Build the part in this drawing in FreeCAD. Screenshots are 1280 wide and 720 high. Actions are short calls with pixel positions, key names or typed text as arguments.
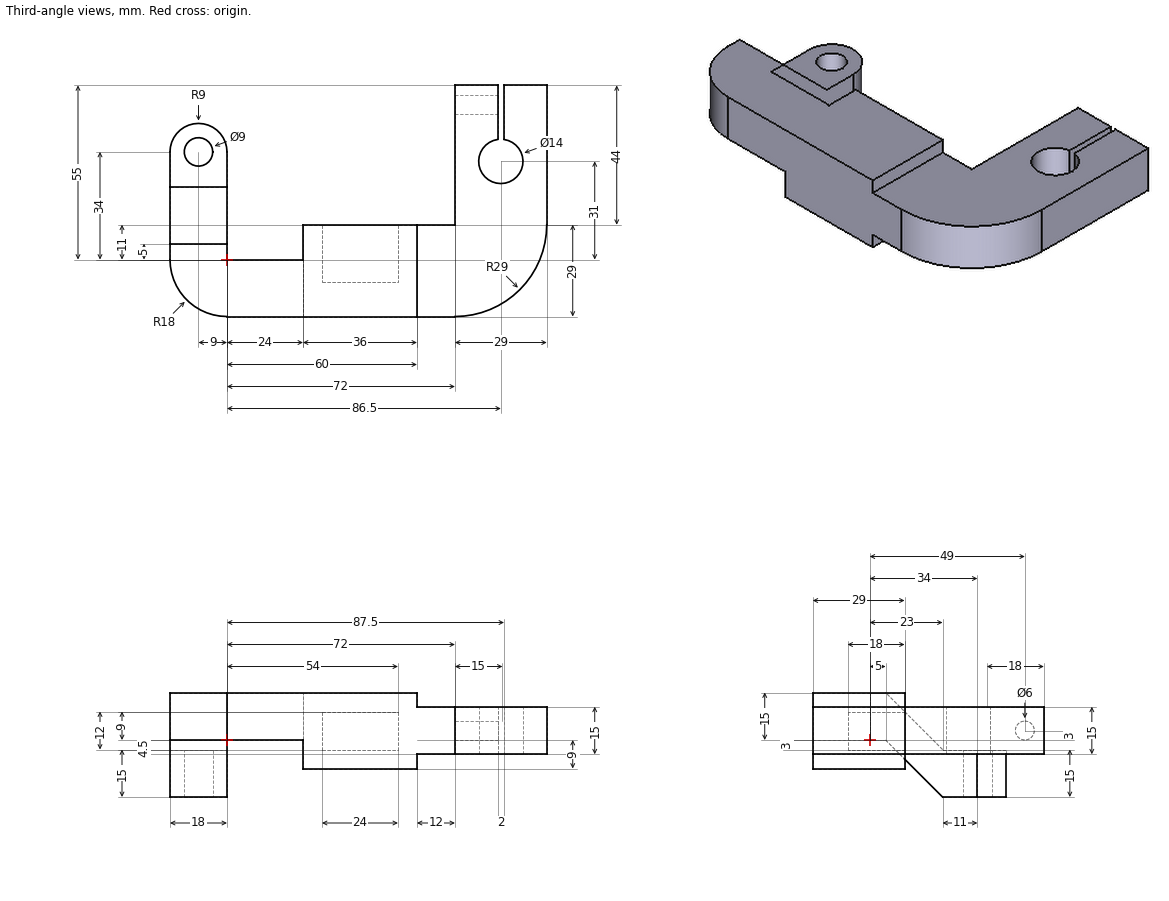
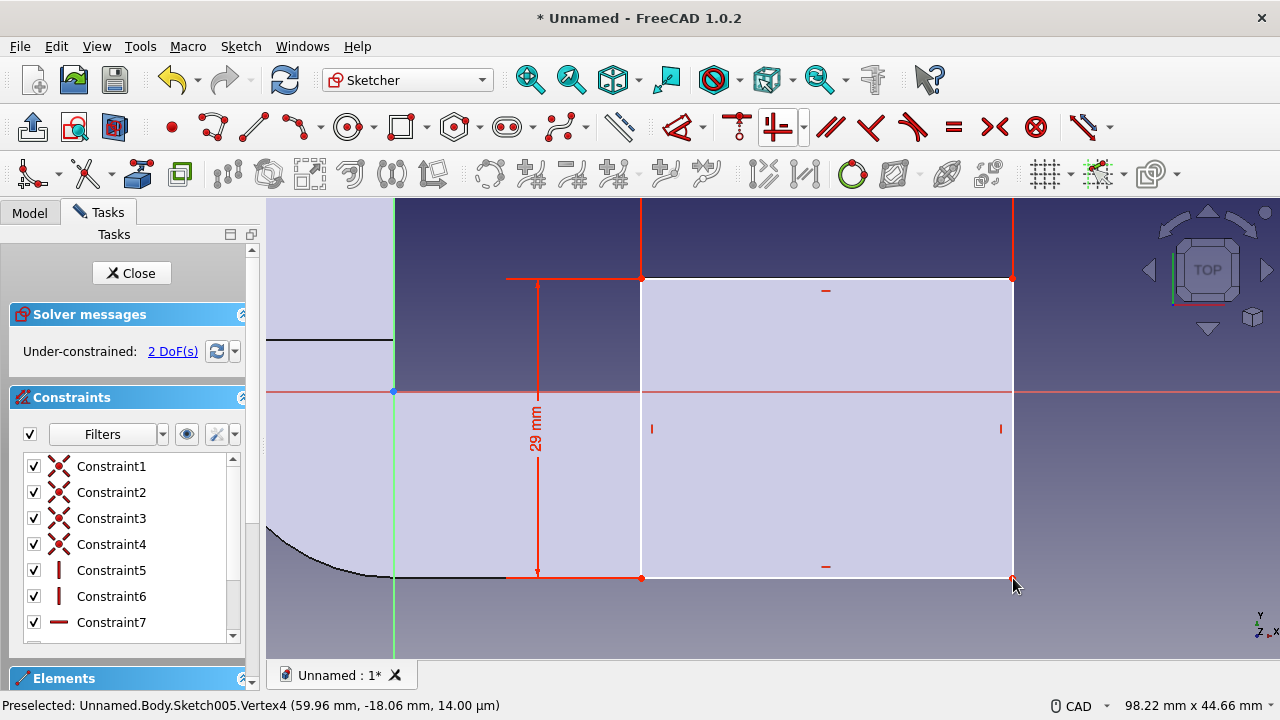
click(676, 128)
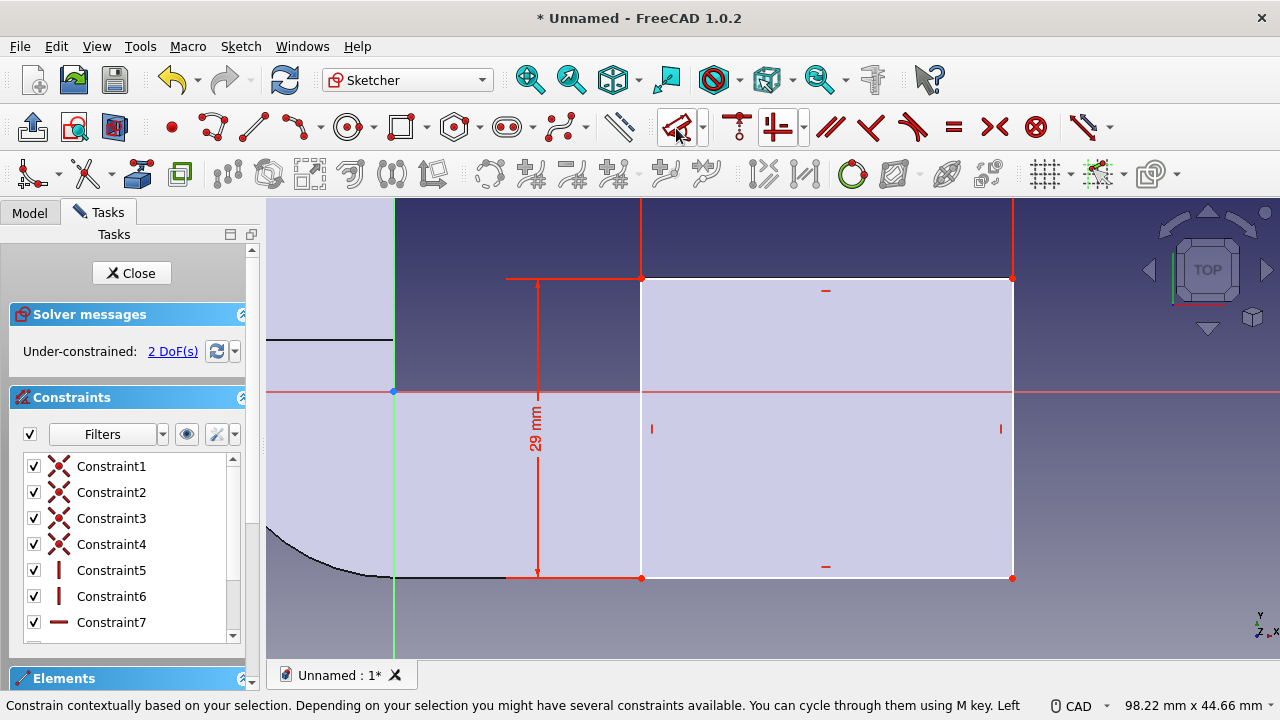
click(641, 279)
click(517, 245)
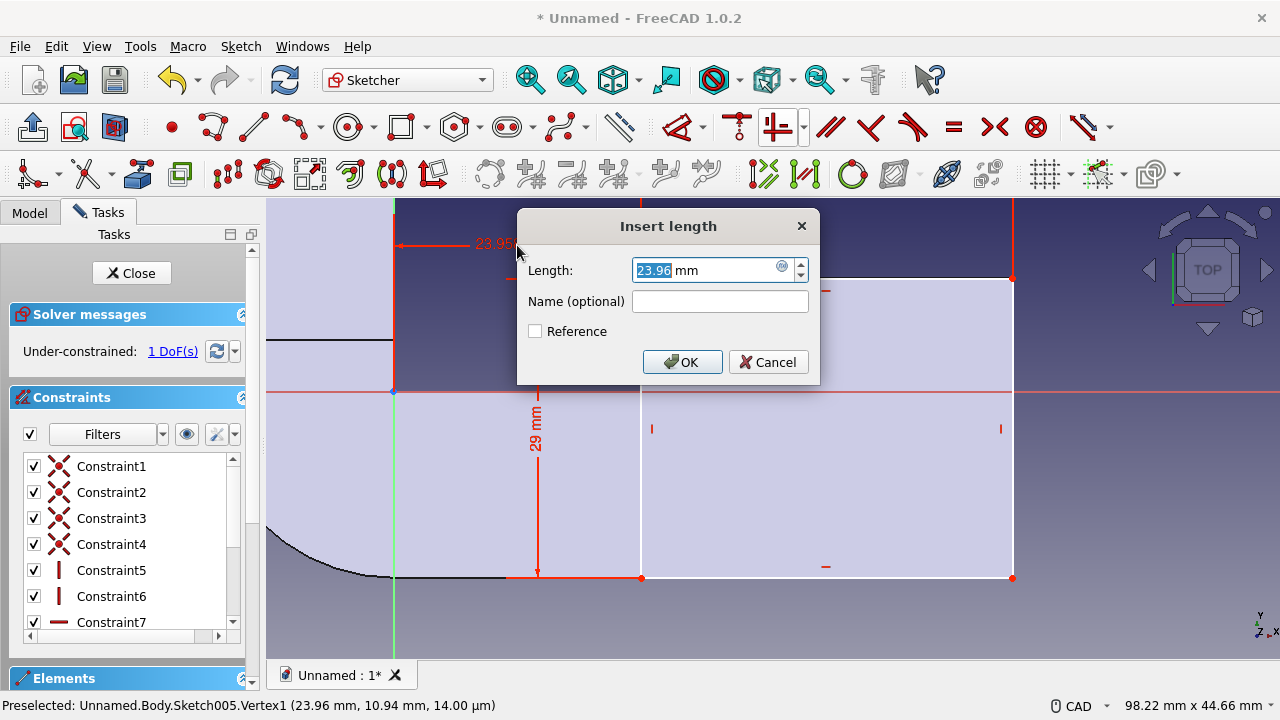
text(24)
key(Return)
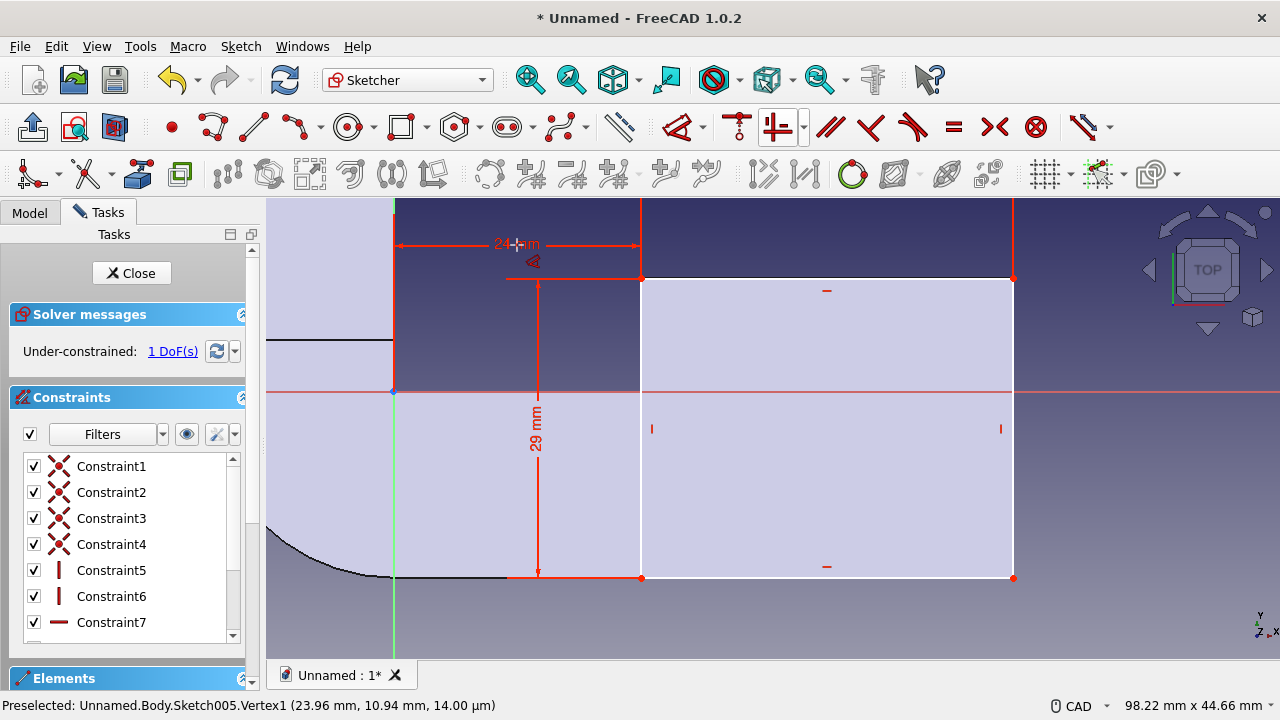
click(641, 279)
click(360, 335)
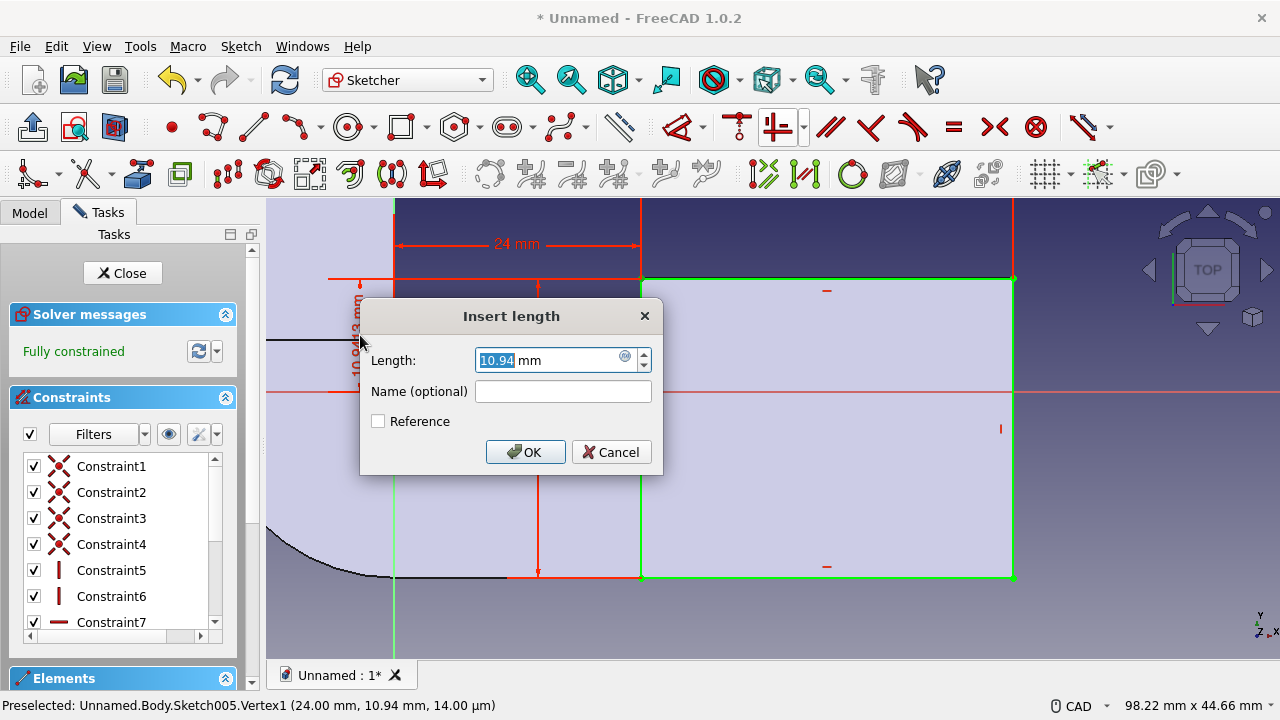
text(11)
key(Return)
key(Escape)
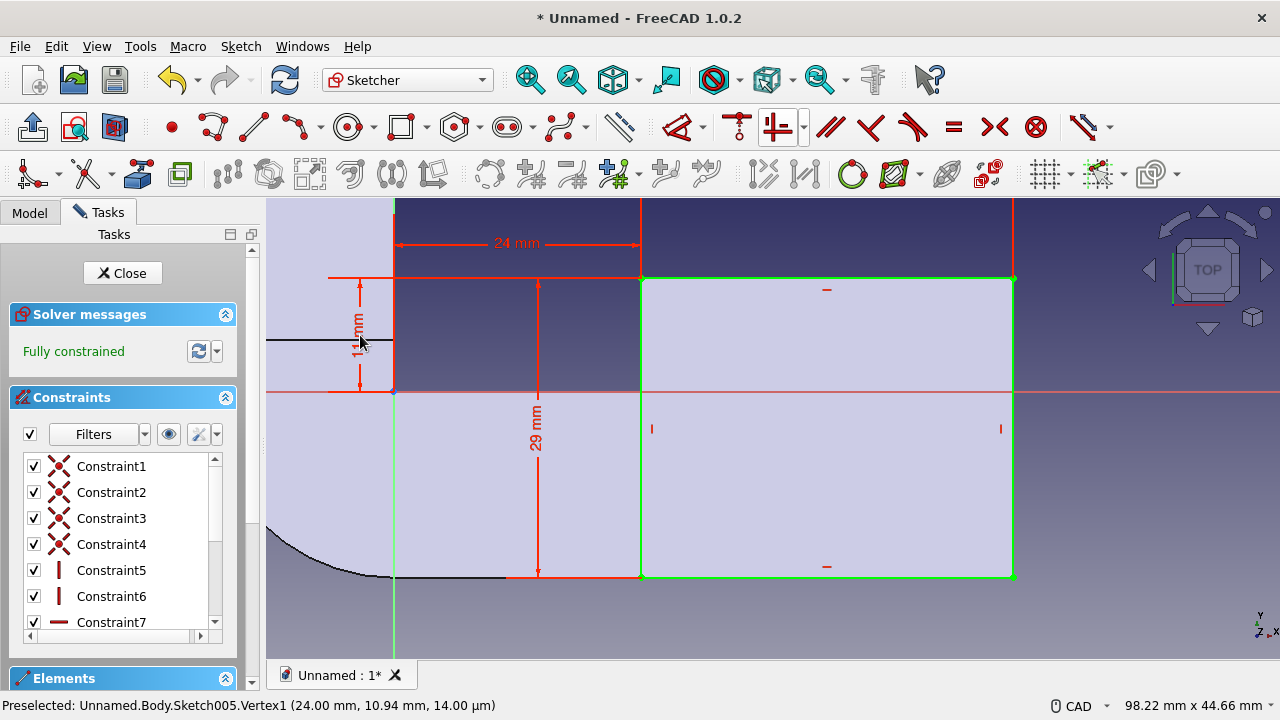
click(123, 273)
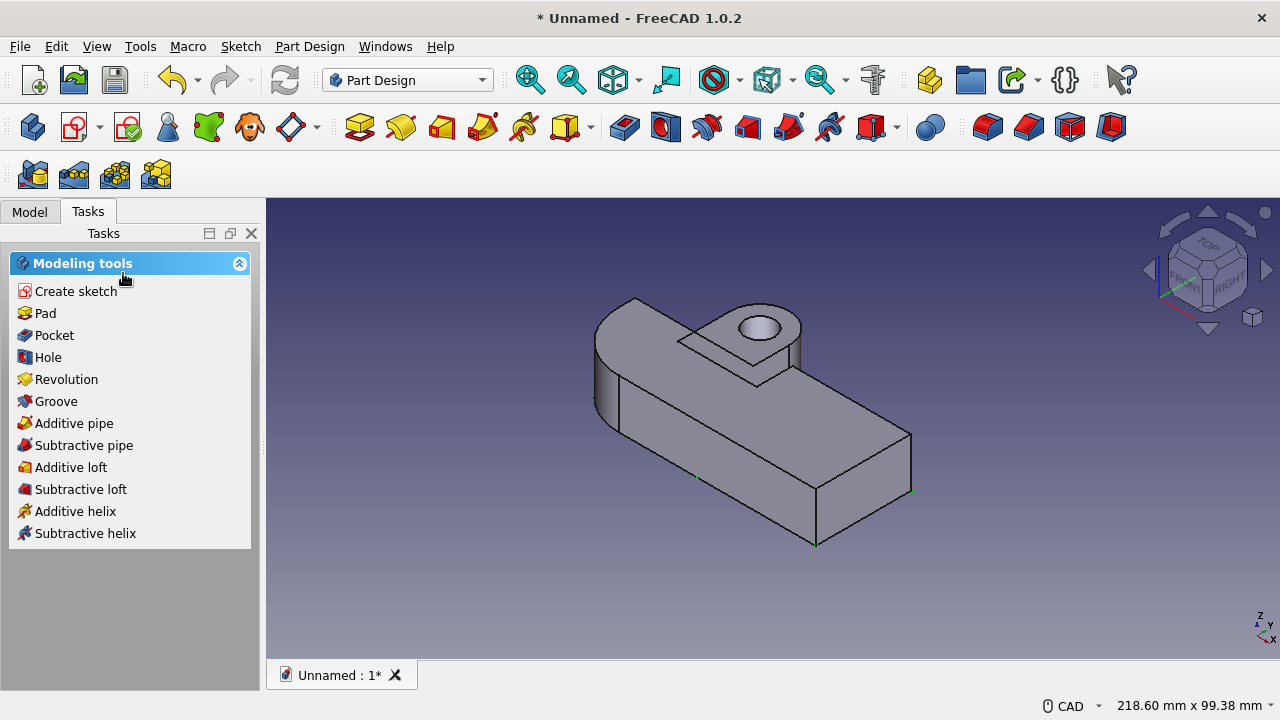
click(360, 128)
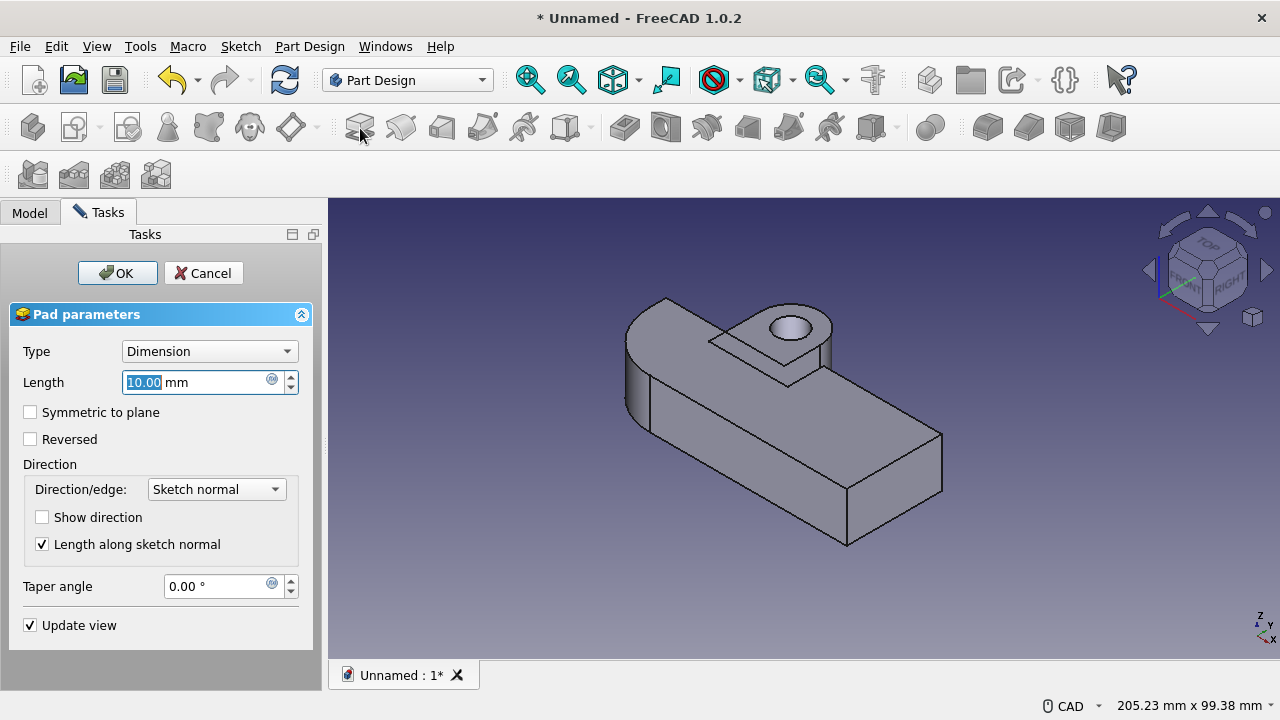
text(9)
key(Tab)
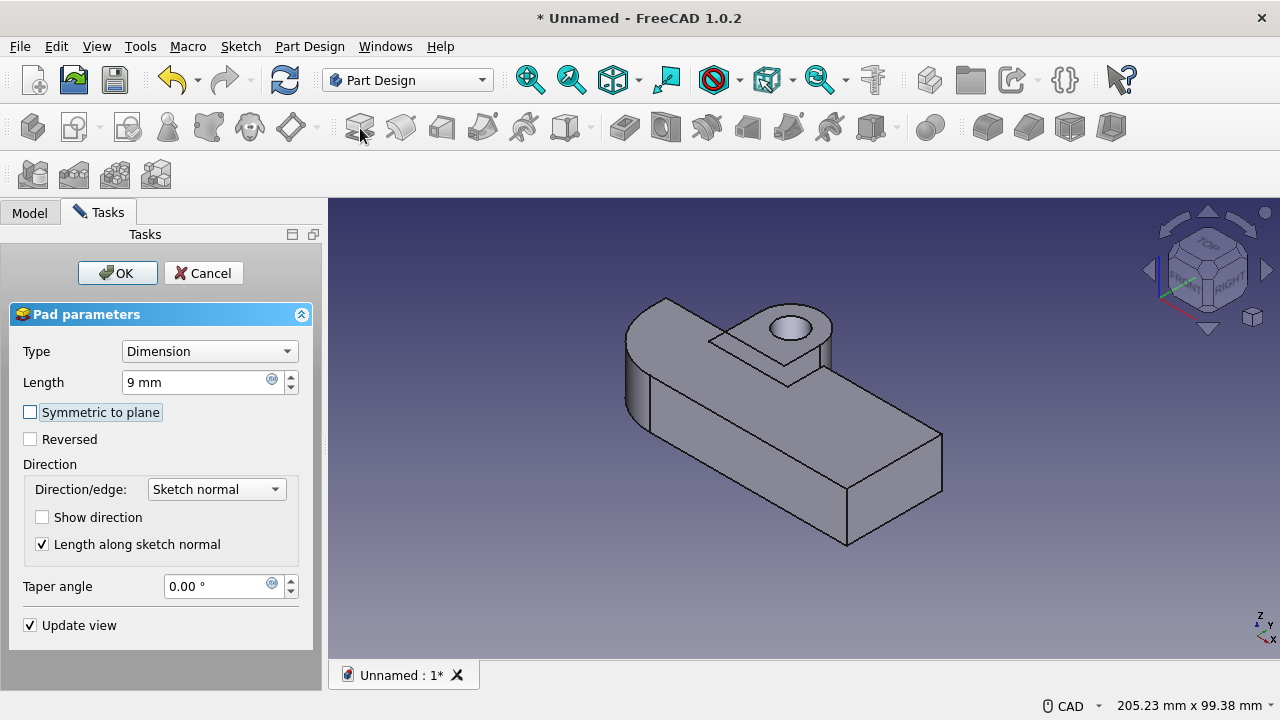
click(31, 439)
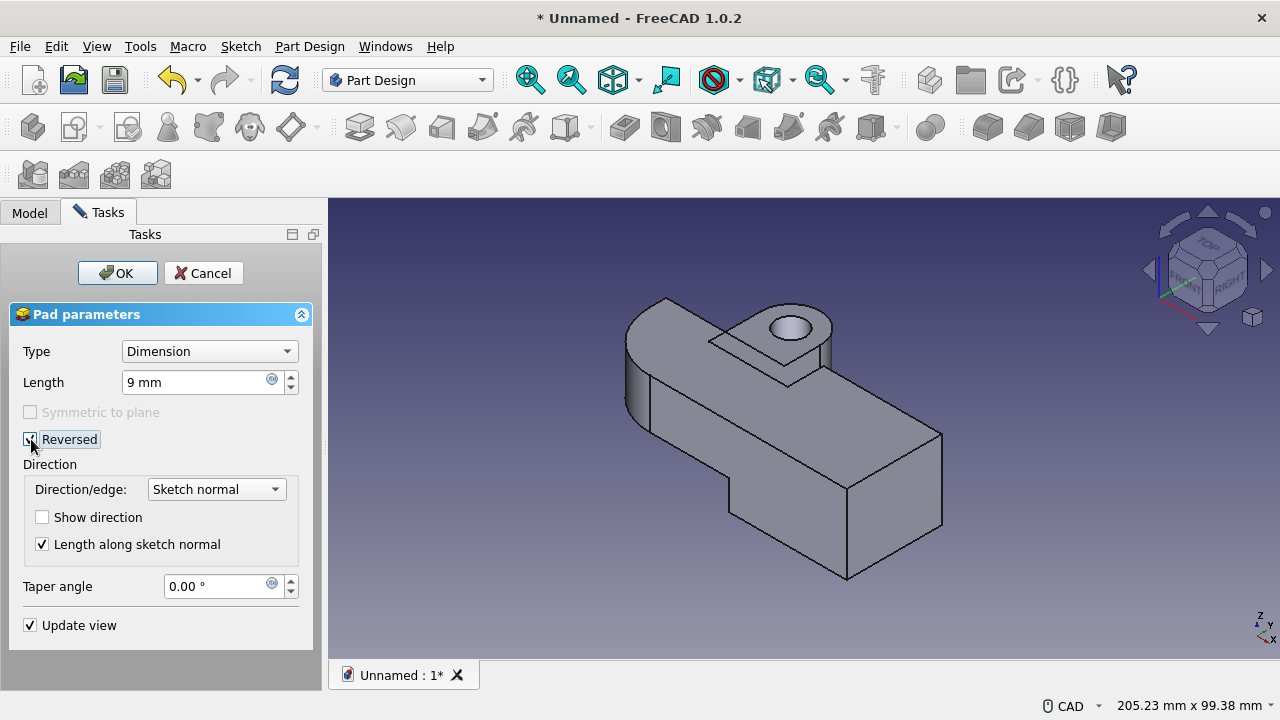
click(118, 273)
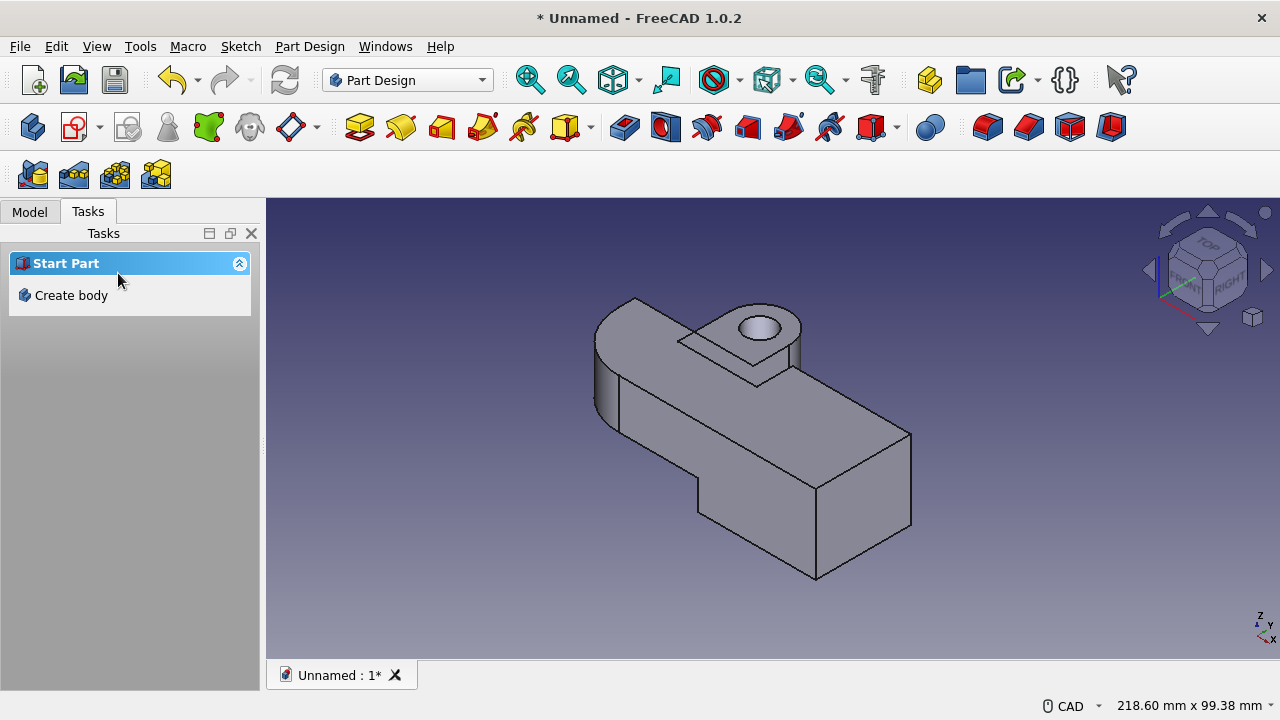
key(4)